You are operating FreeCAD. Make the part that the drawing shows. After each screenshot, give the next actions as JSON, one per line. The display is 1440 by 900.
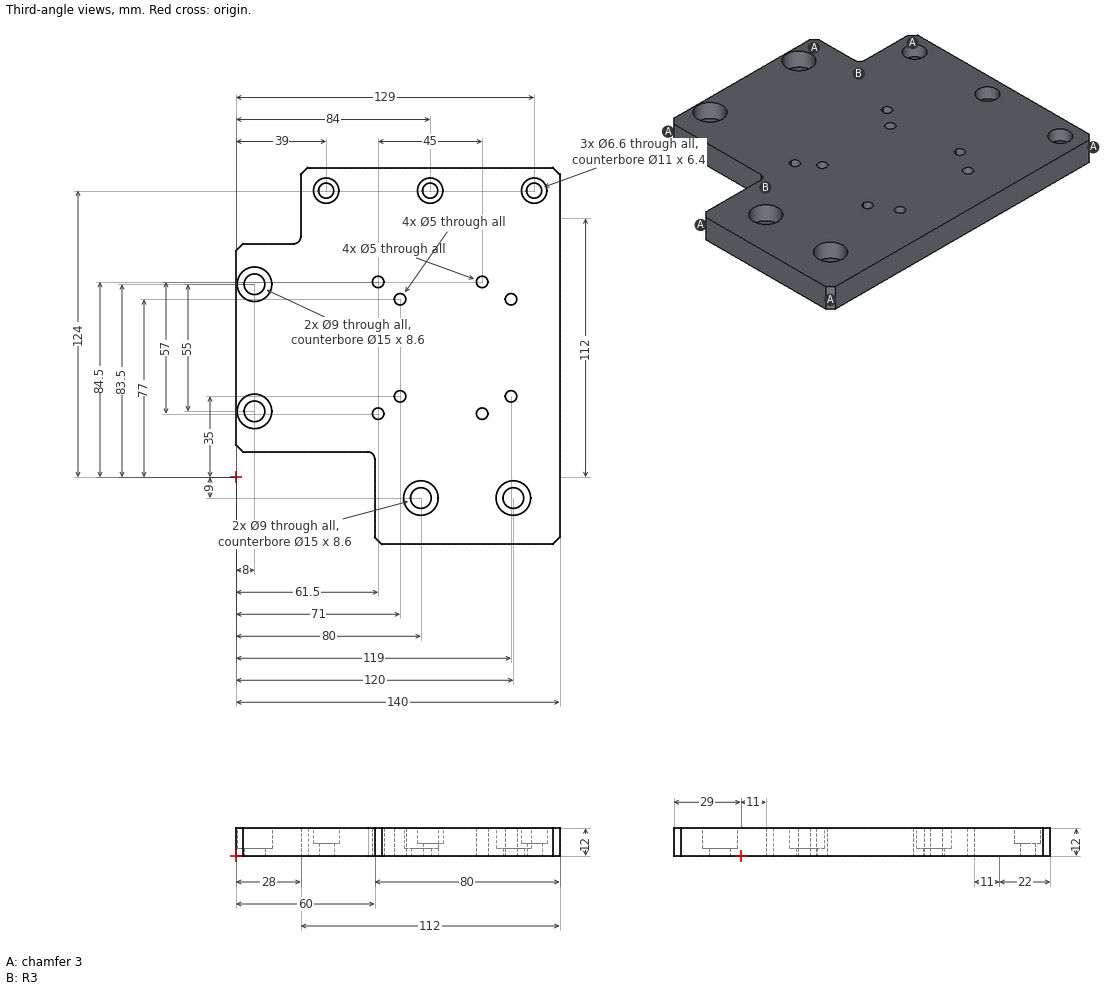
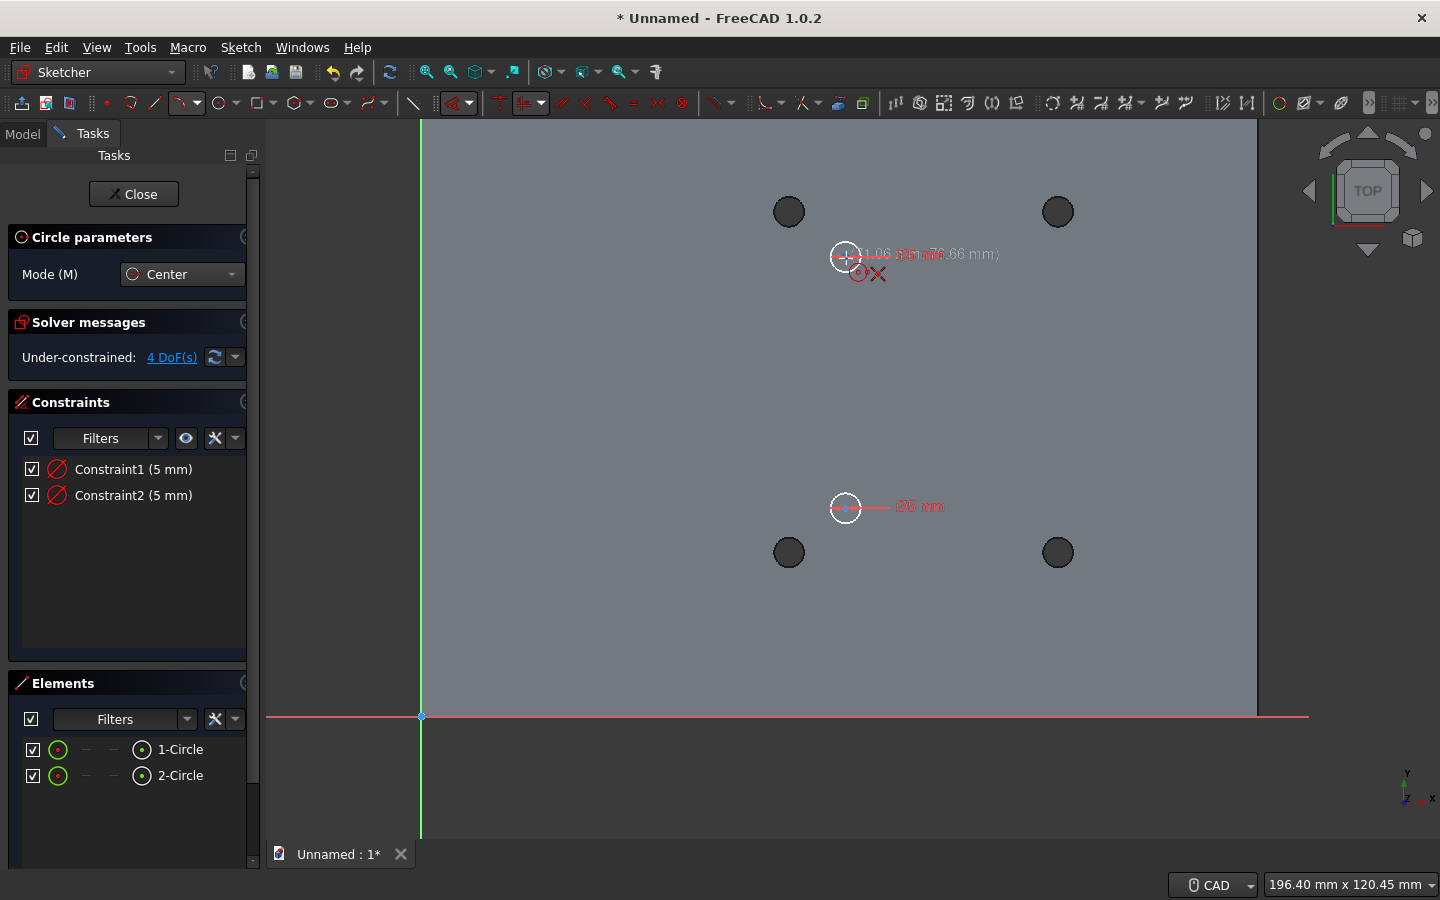
{"action": "scroll", "coordinate": [1133, 508], "scroll_direction": "up", "scroll_amount": 3}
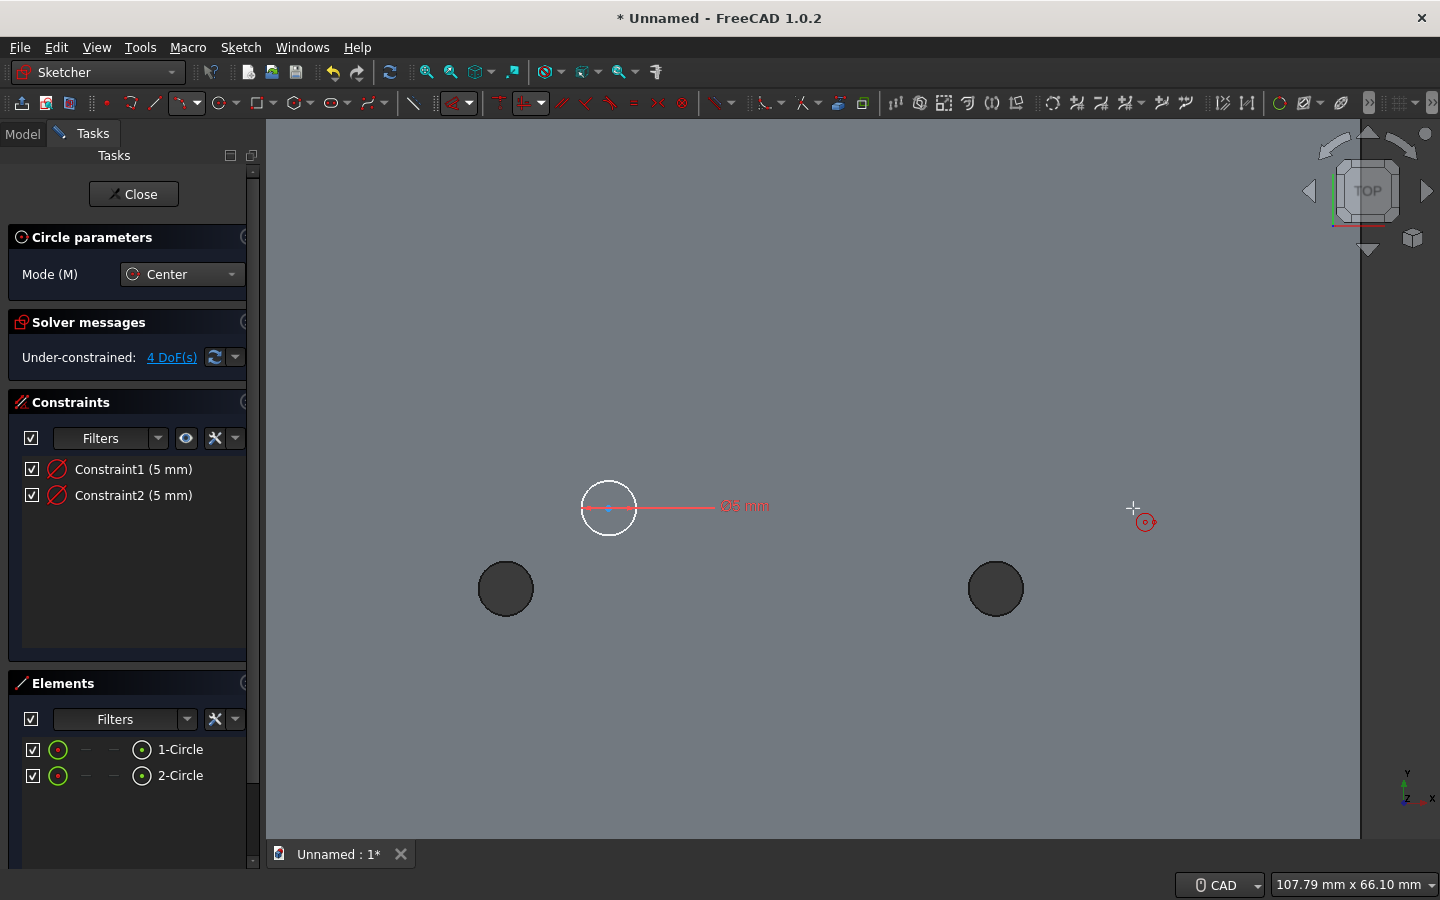
{"action": "left_click", "coordinate": [1132, 507]}
{"action": "mouse_move", "coordinate": [1151, 488]}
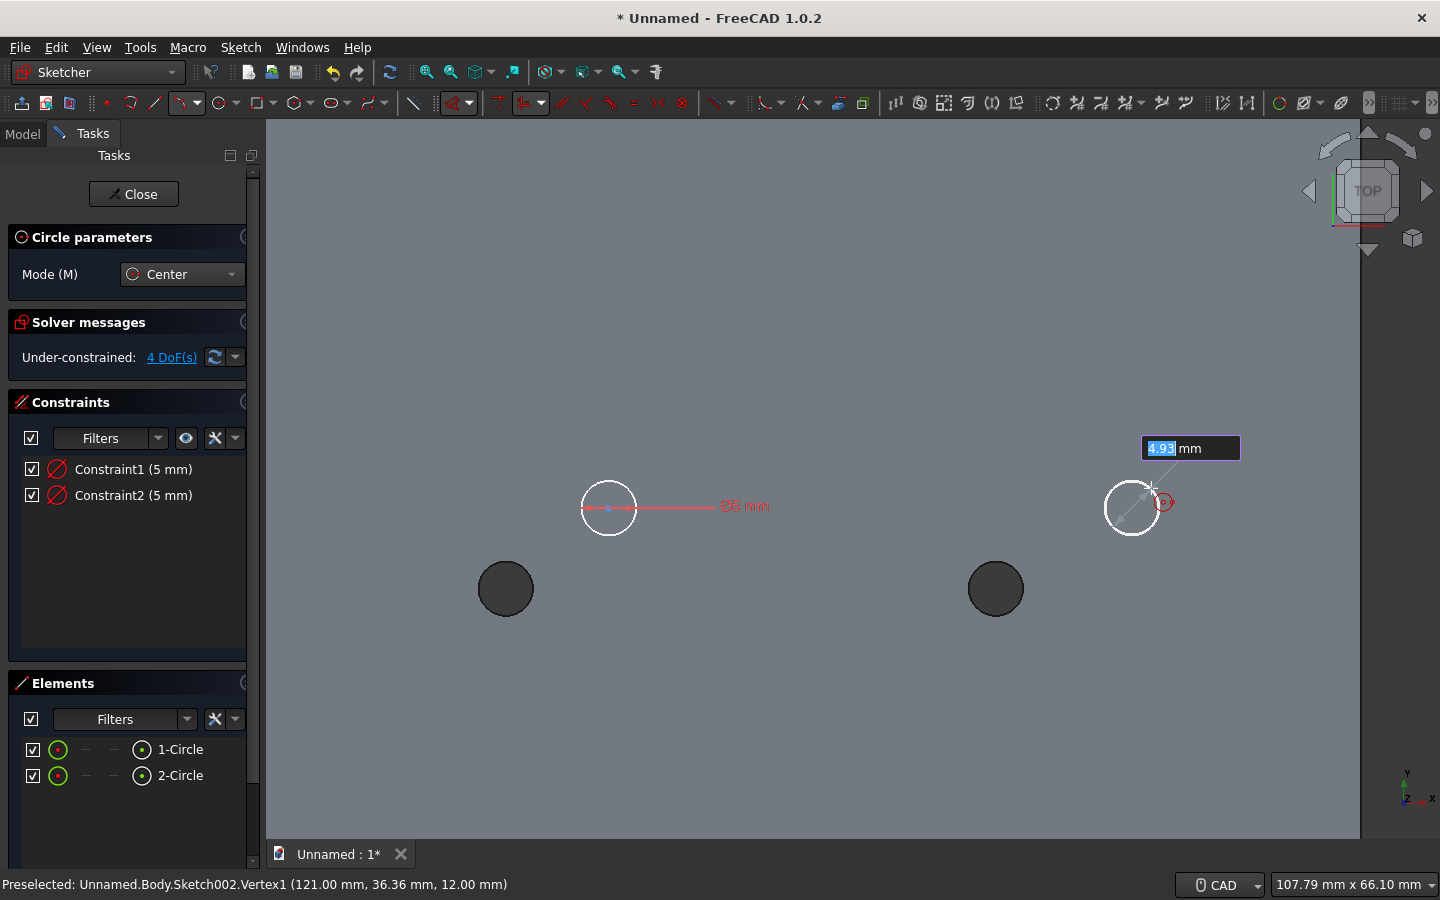
{"action": "type", "text": "5"}
{"action": "key", "text": "Return"}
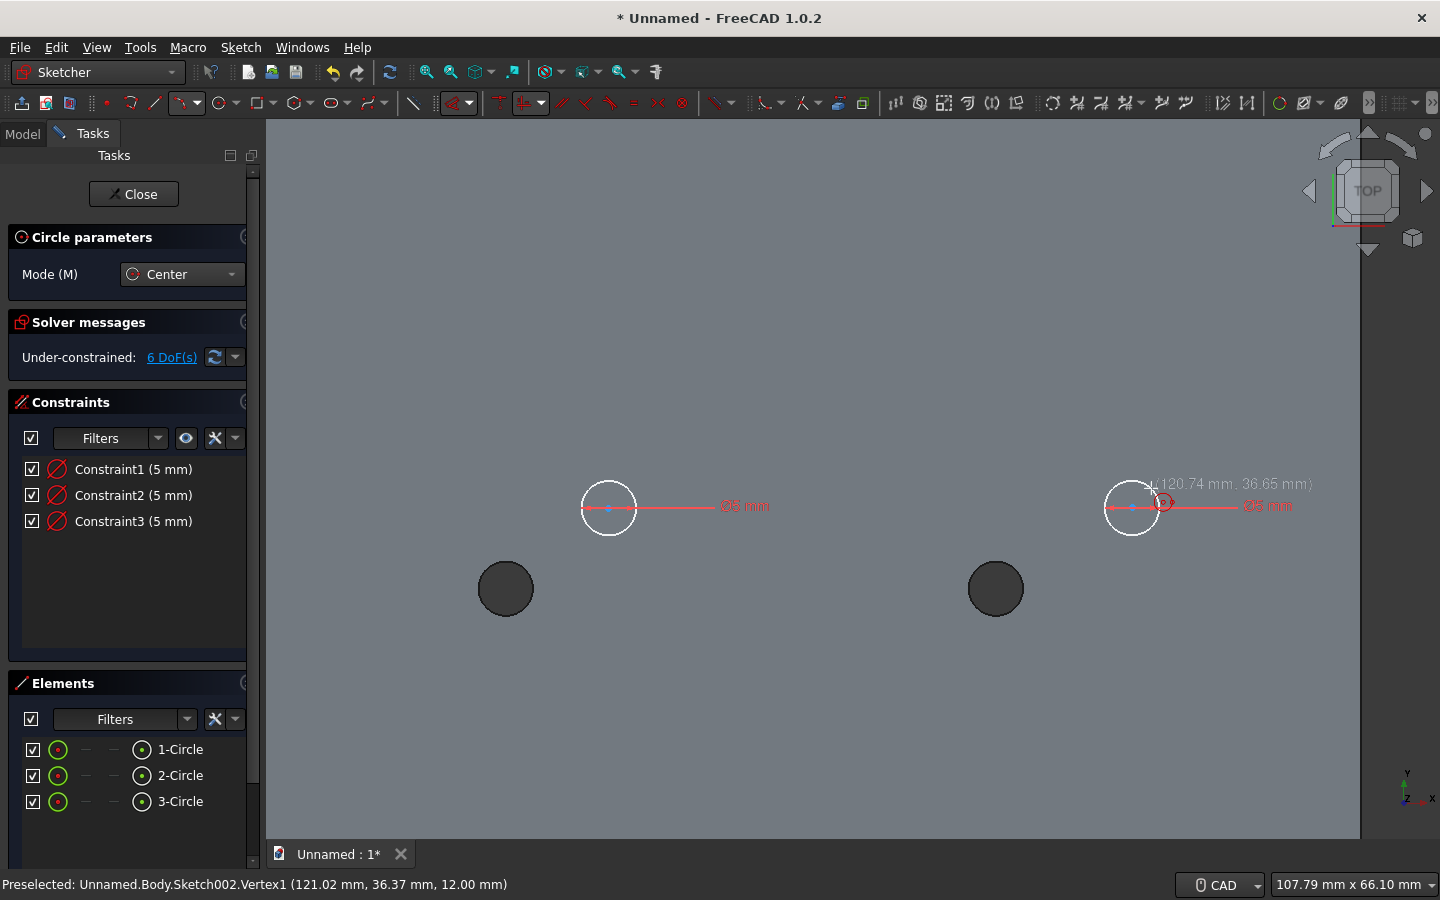
{"action": "scroll", "coordinate": [1133, 508], "scroll_direction": "down", "scroll_amount": 3}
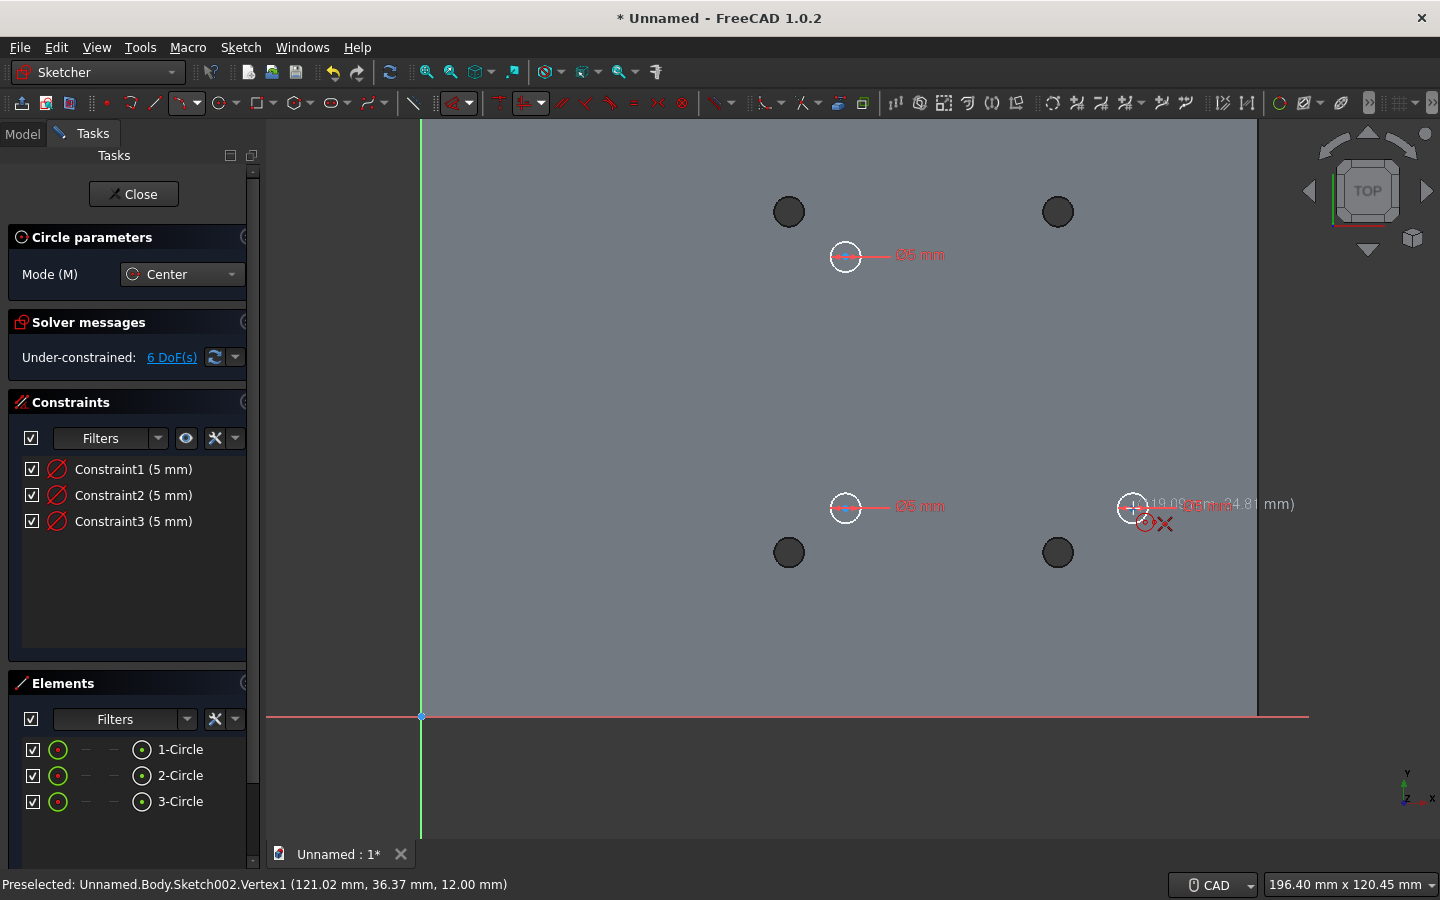
{"action": "scroll", "coordinate": [1133, 257], "scroll_direction": "up", "scroll_amount": 3}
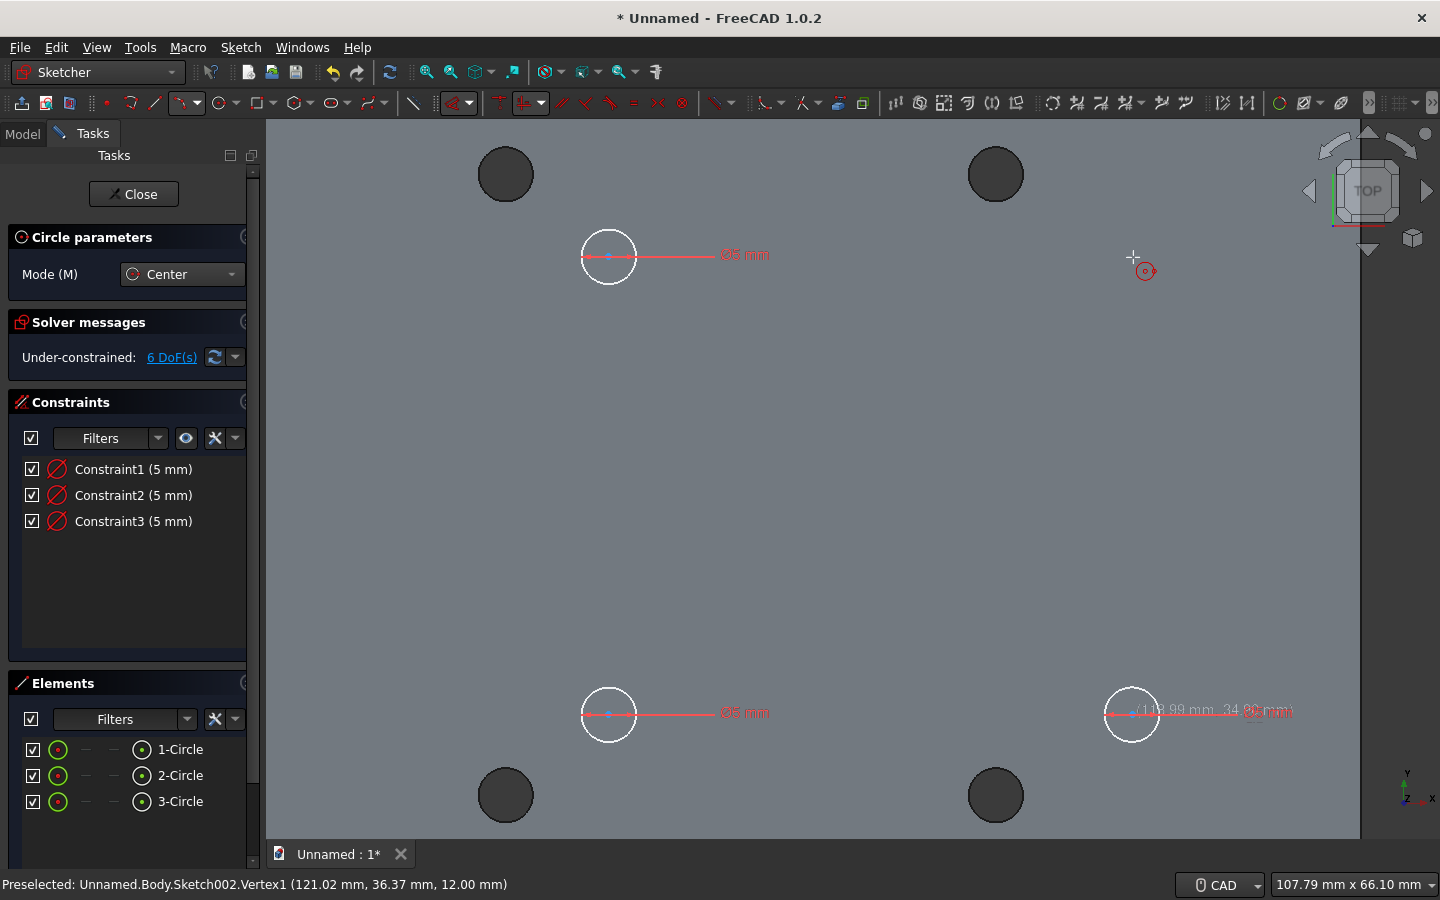
{"action": "left_click", "coordinate": [1132, 256]}
{"action": "mouse_move", "coordinate": [1151, 237]}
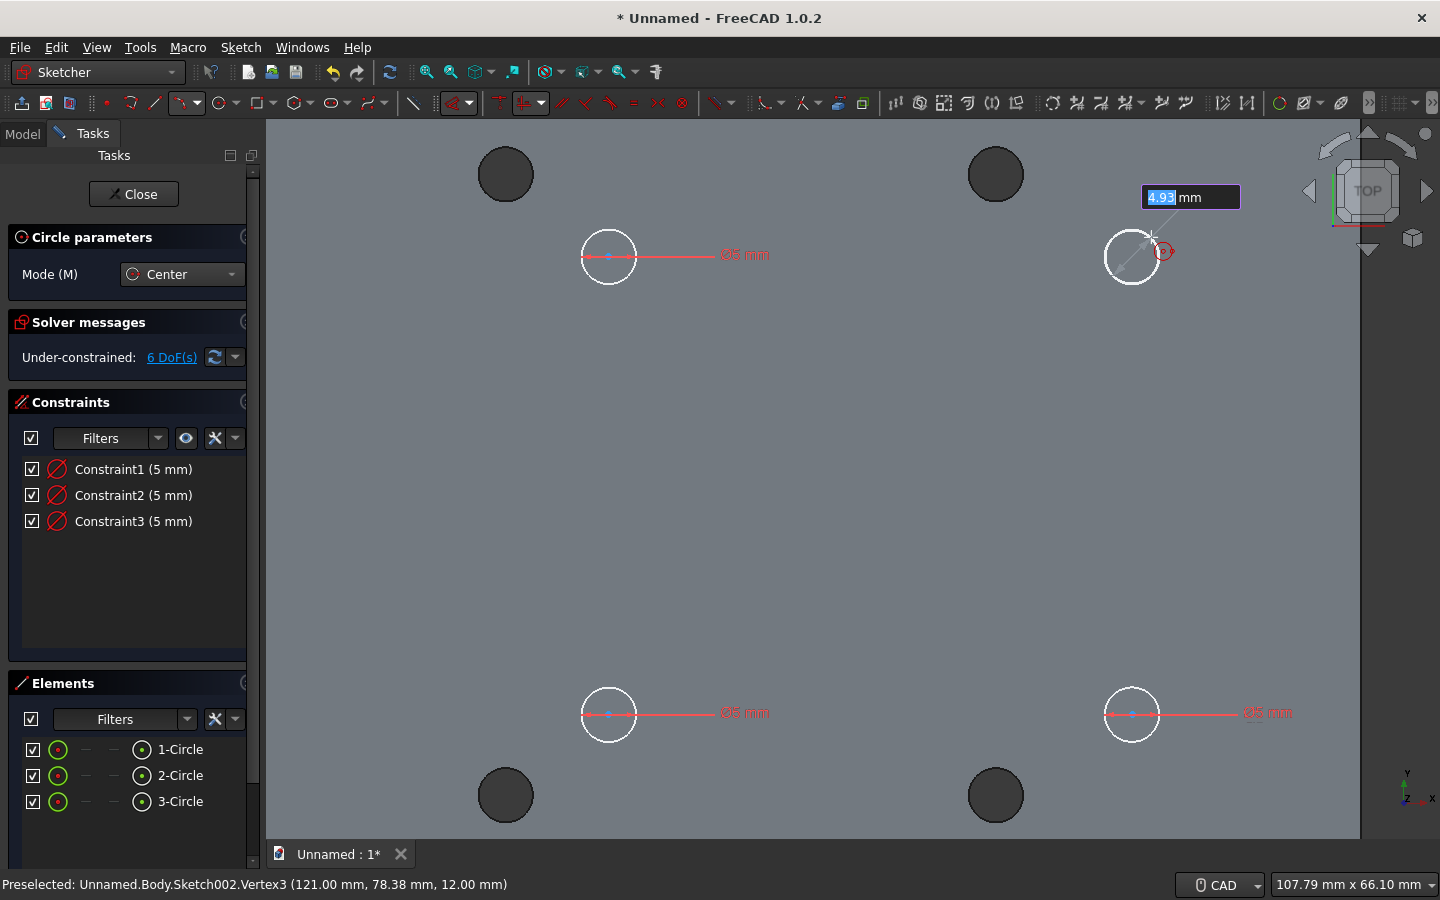
{"action": "type", "text": "5"}
{"action": "key", "text": "Return"}
{"action": "key", "text": "Escape"}